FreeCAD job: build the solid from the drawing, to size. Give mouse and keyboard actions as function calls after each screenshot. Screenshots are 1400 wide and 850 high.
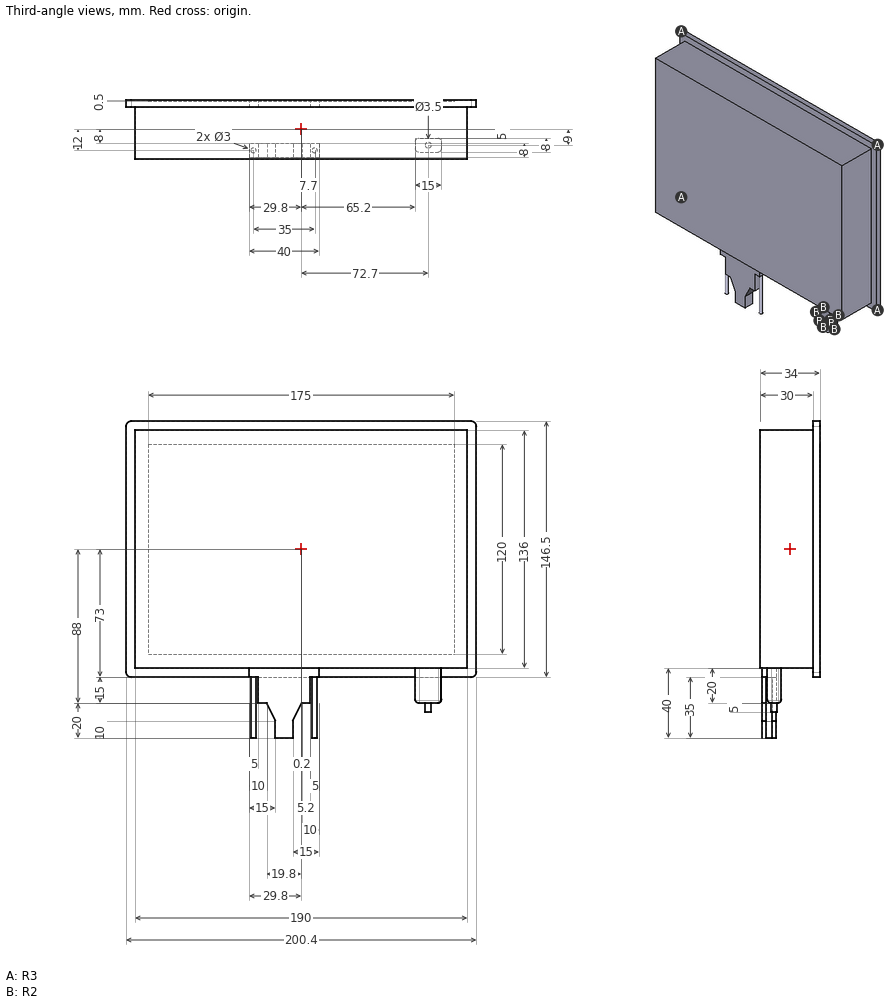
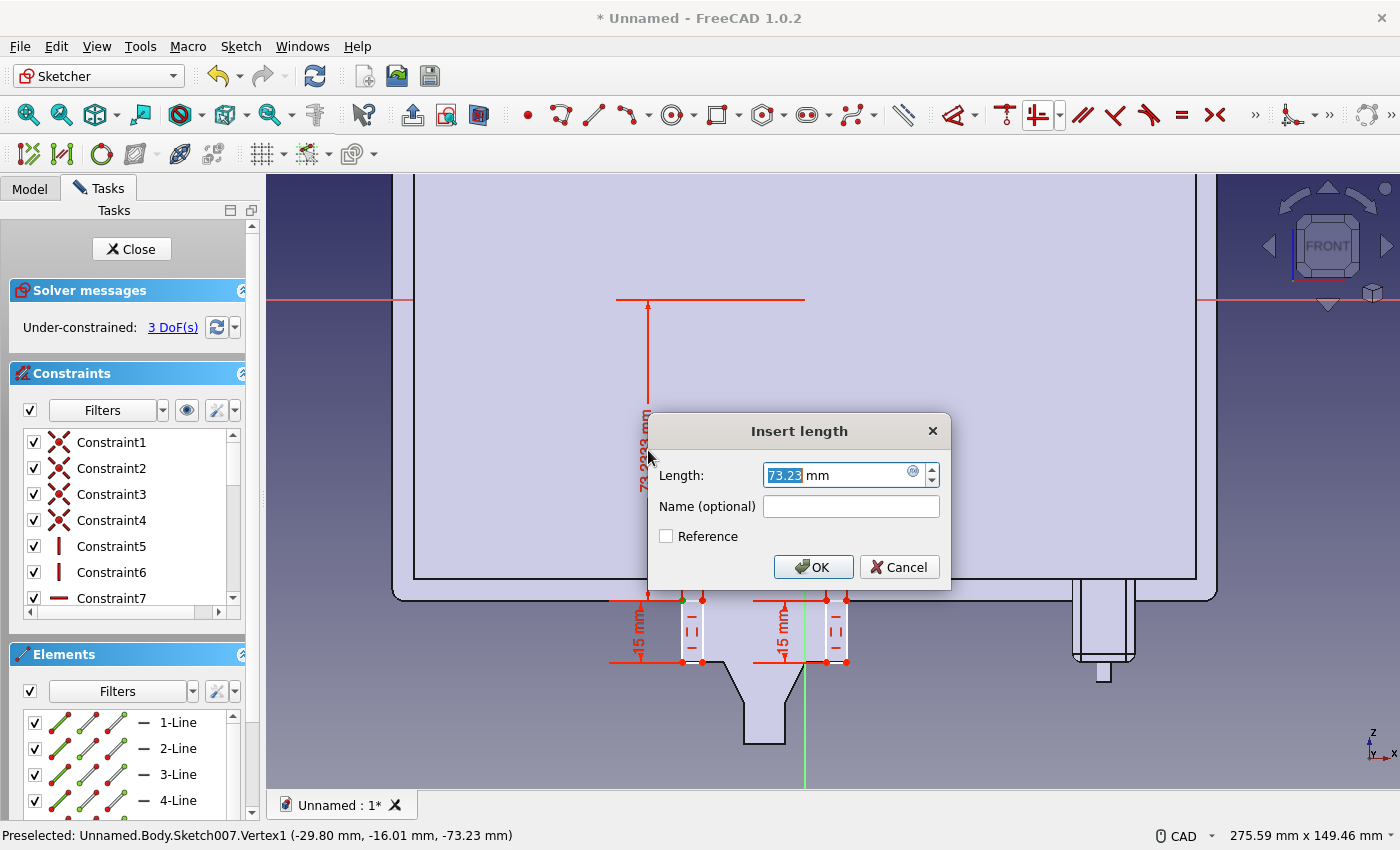
text(73)
key(Return)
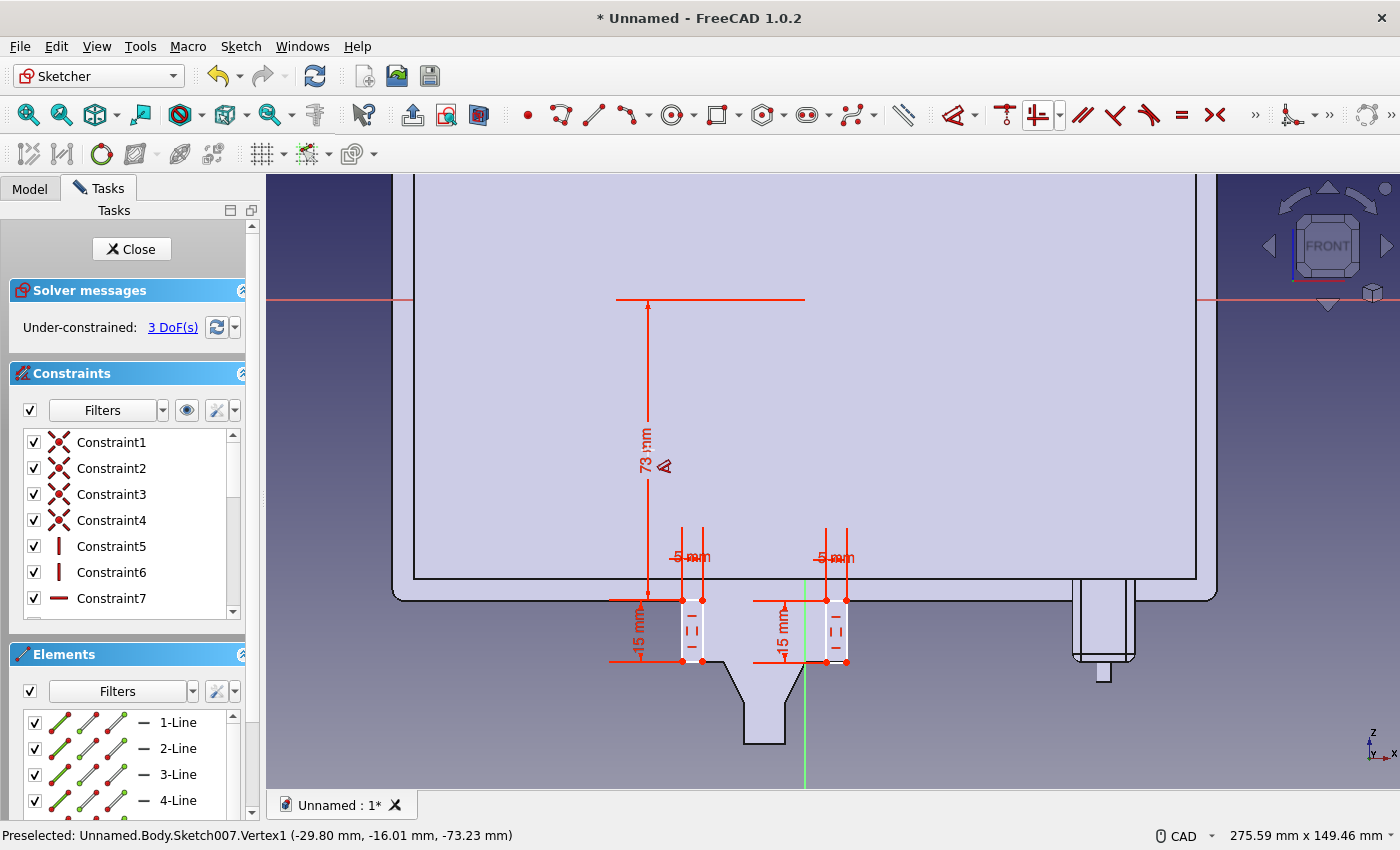
click(826, 601)
click(860, 450)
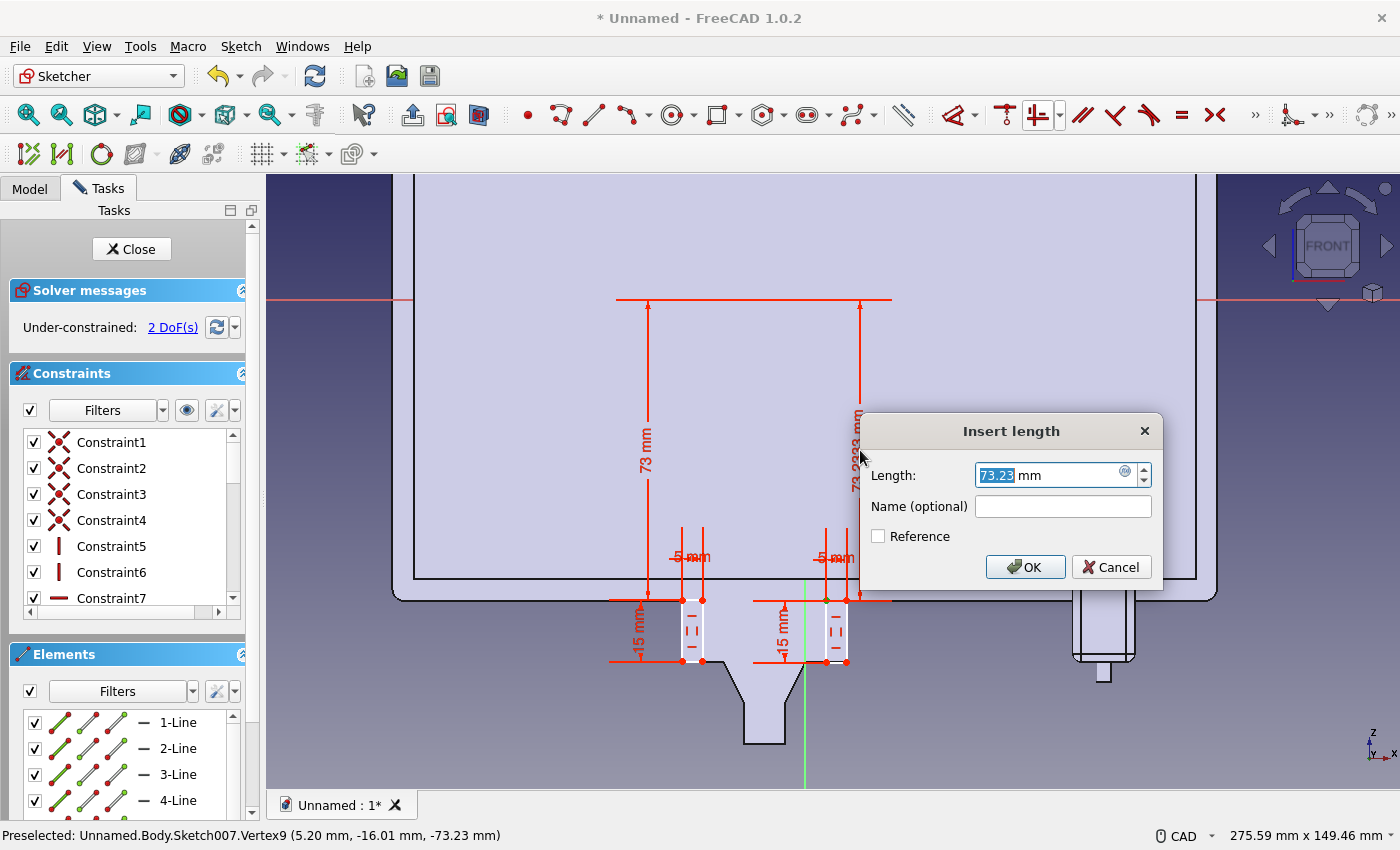
text(73)
key(Return)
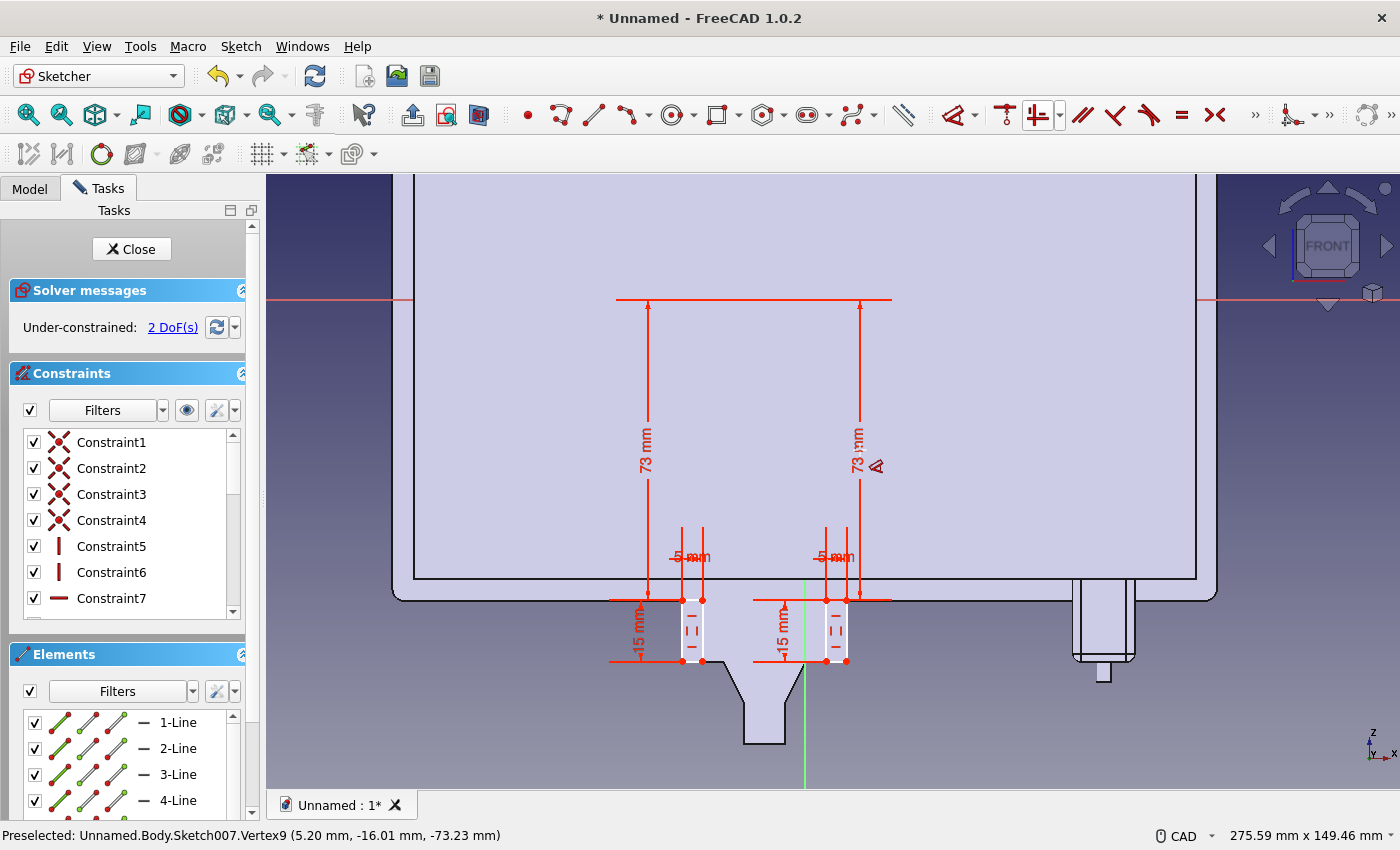
scroll(826, 600, up, 4)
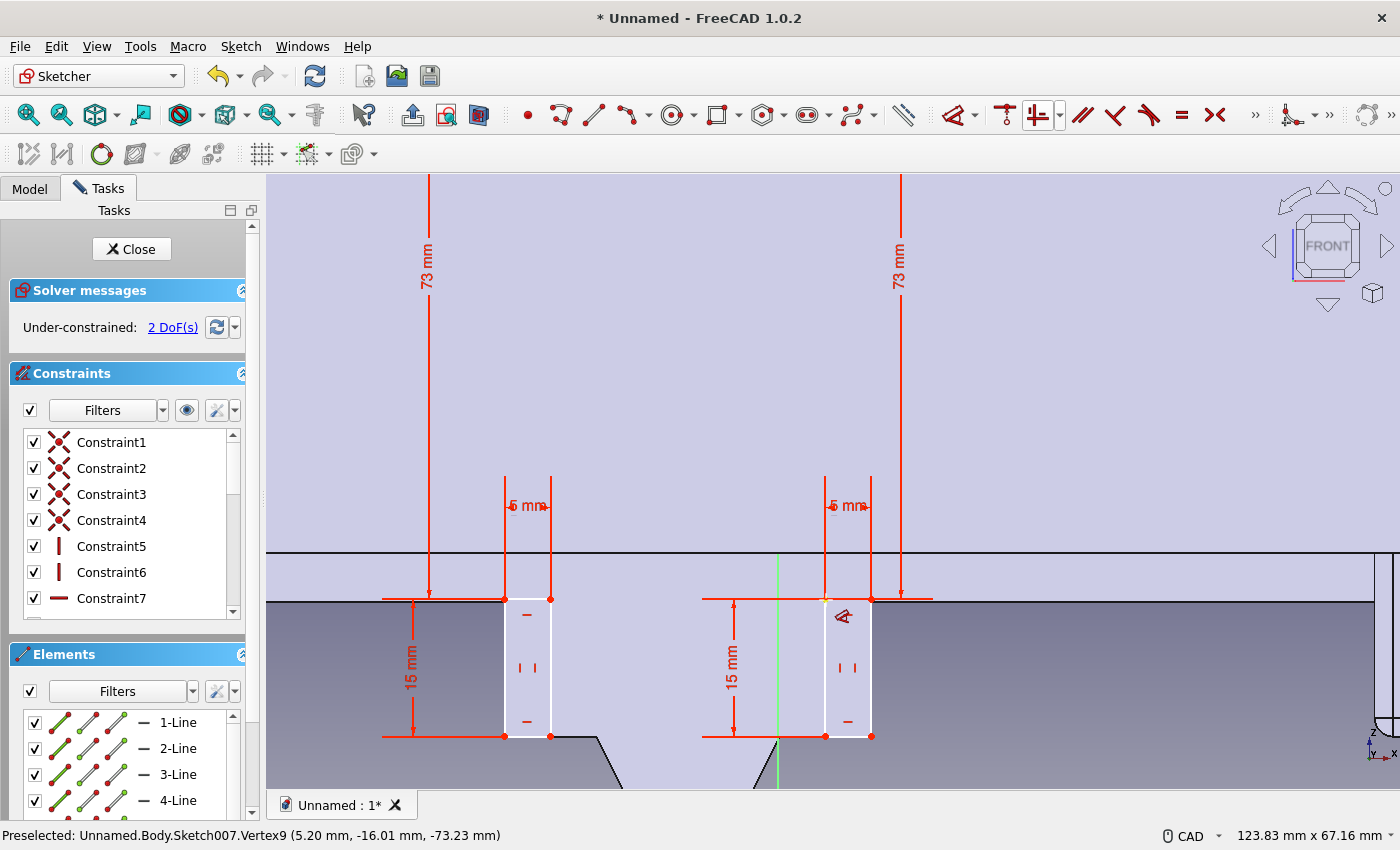
click(825, 599)
click(802, 633)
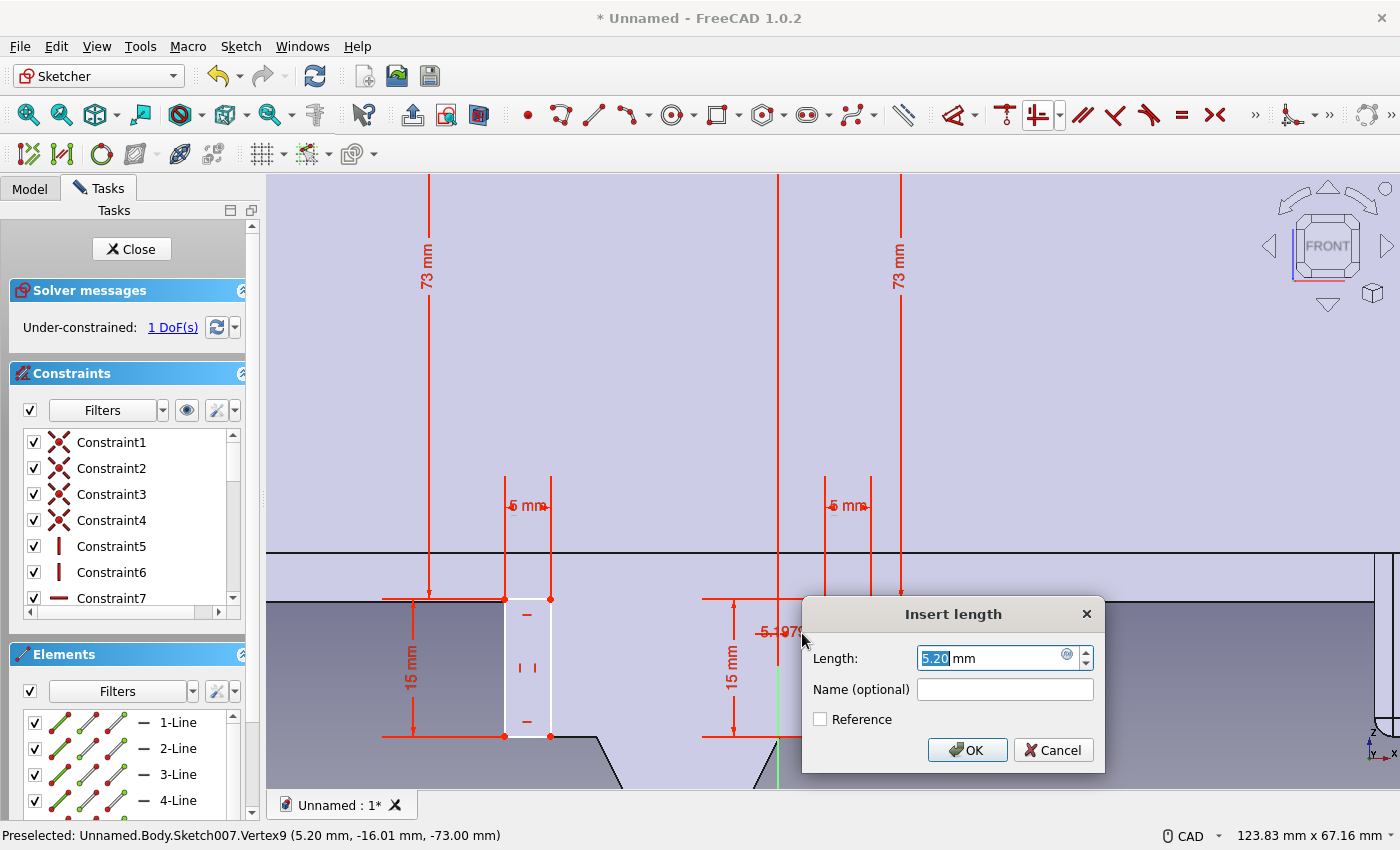
text(5.2)
key(Return)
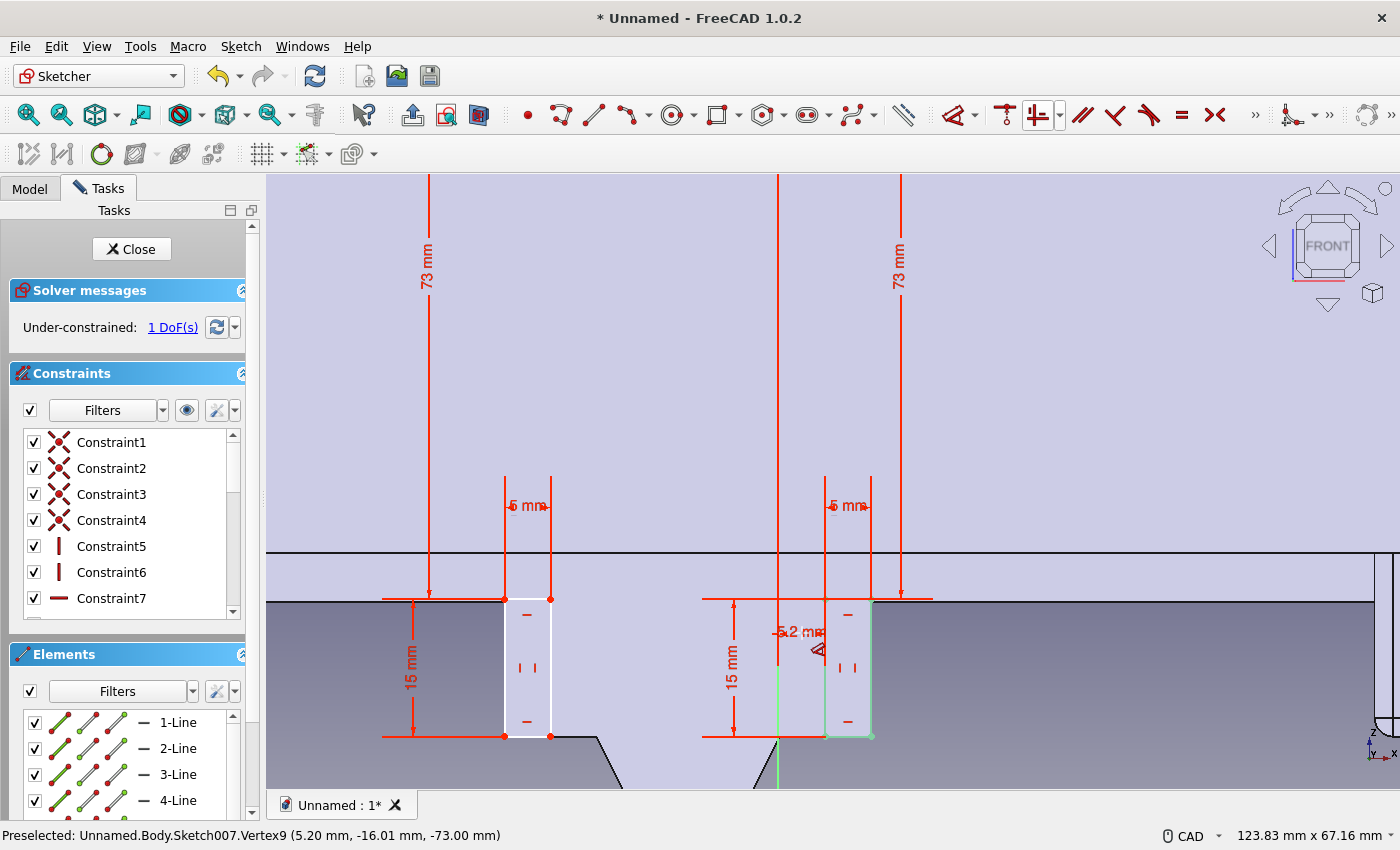
click(505, 599)
click(641, 633)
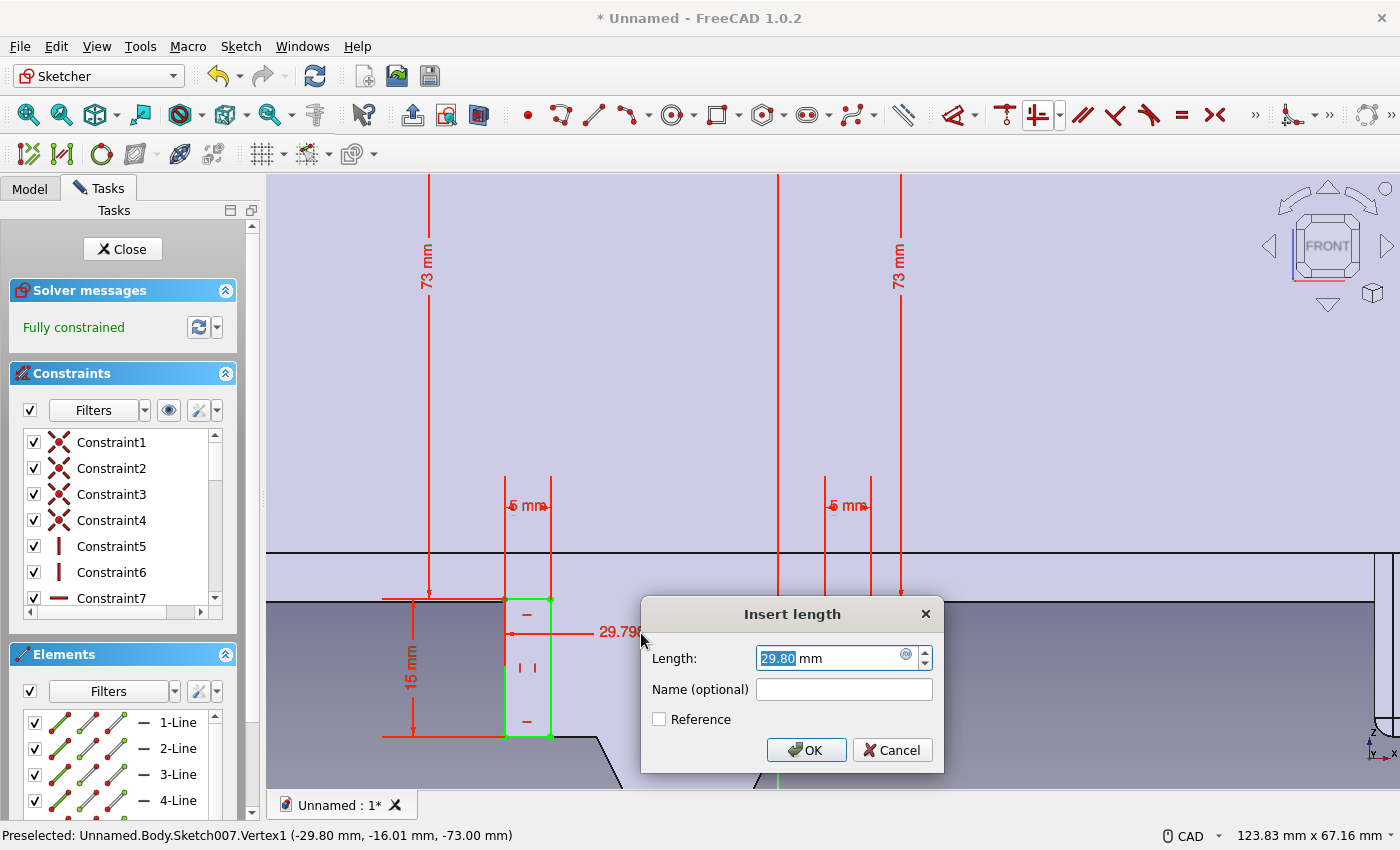
text(29.8)
key(Return)
key(Escape)